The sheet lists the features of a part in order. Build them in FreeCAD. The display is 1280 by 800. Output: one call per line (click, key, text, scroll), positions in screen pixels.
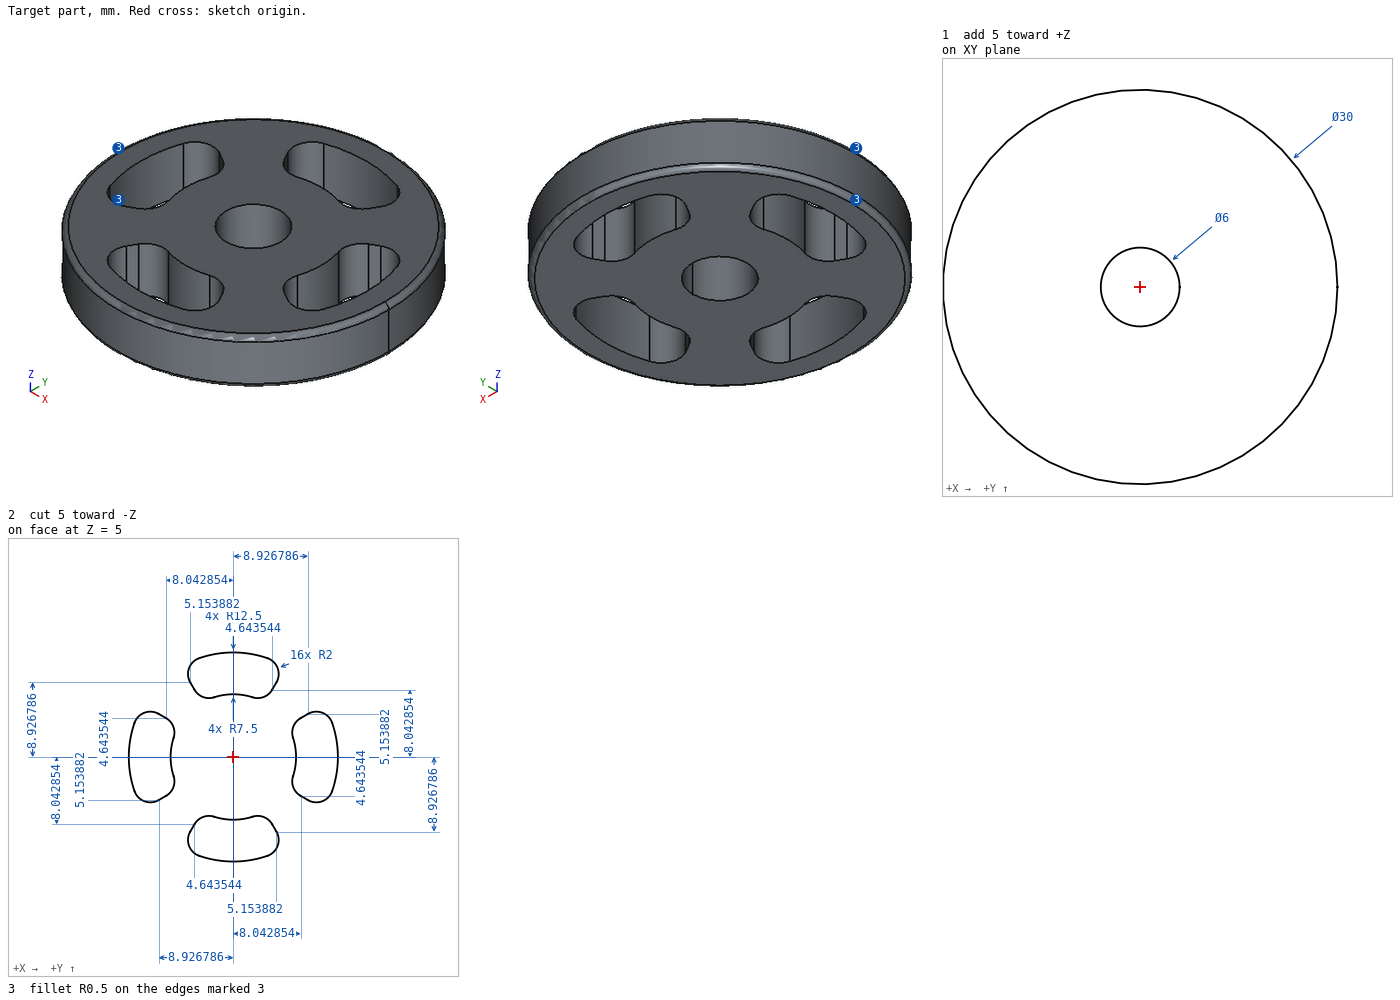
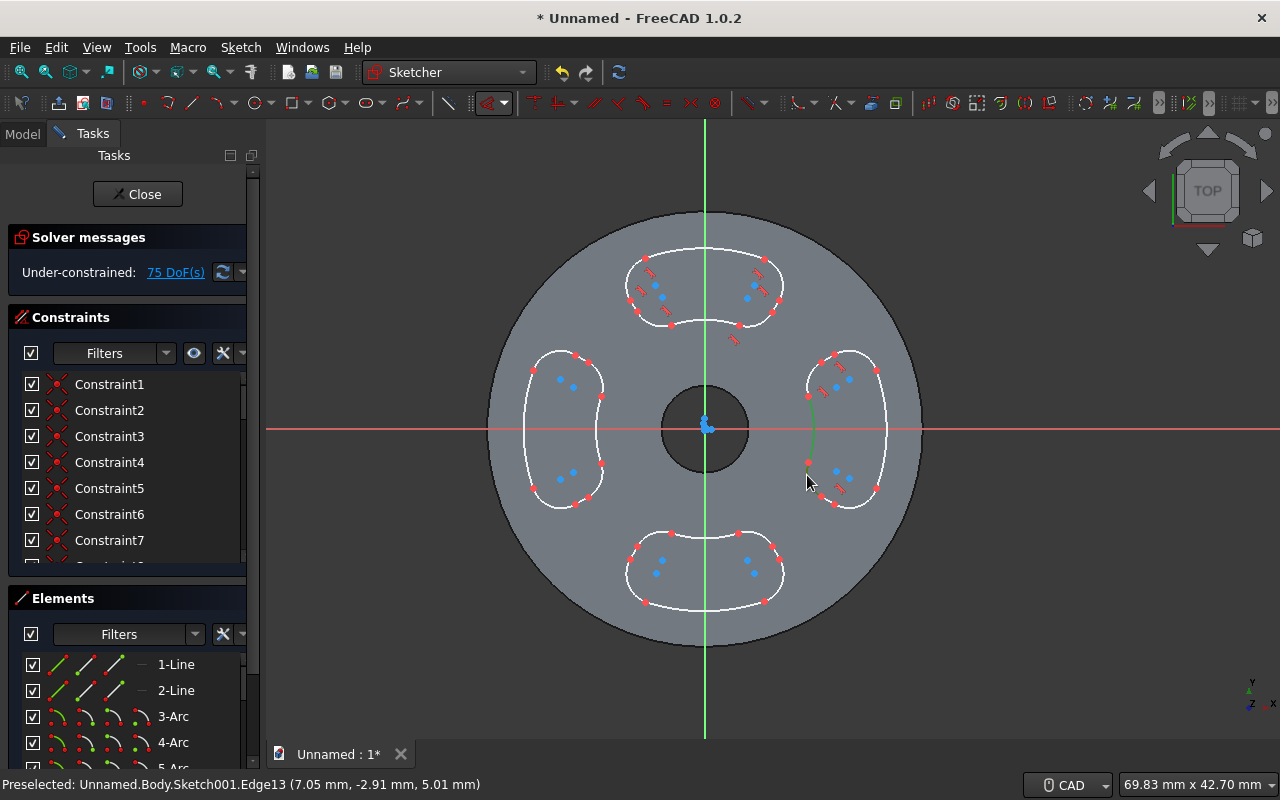
click(644, 104)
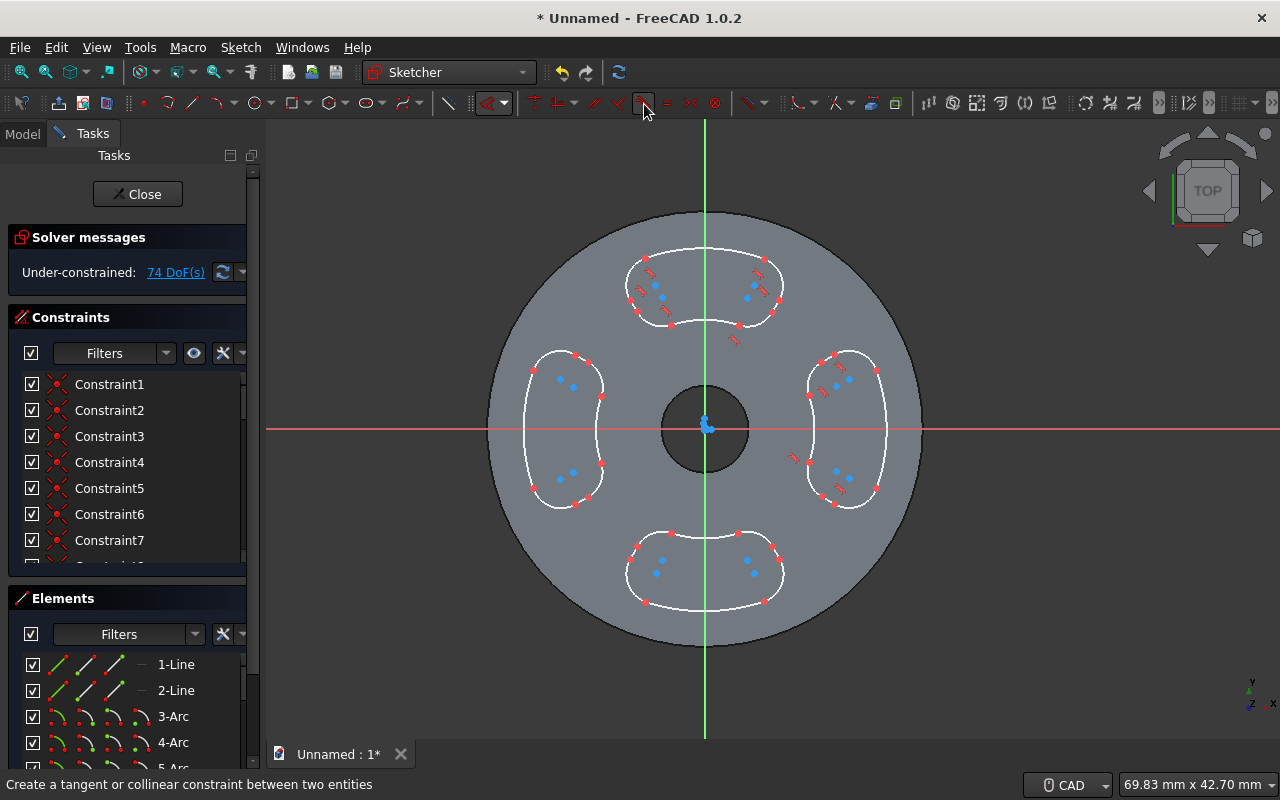
click(849, 508)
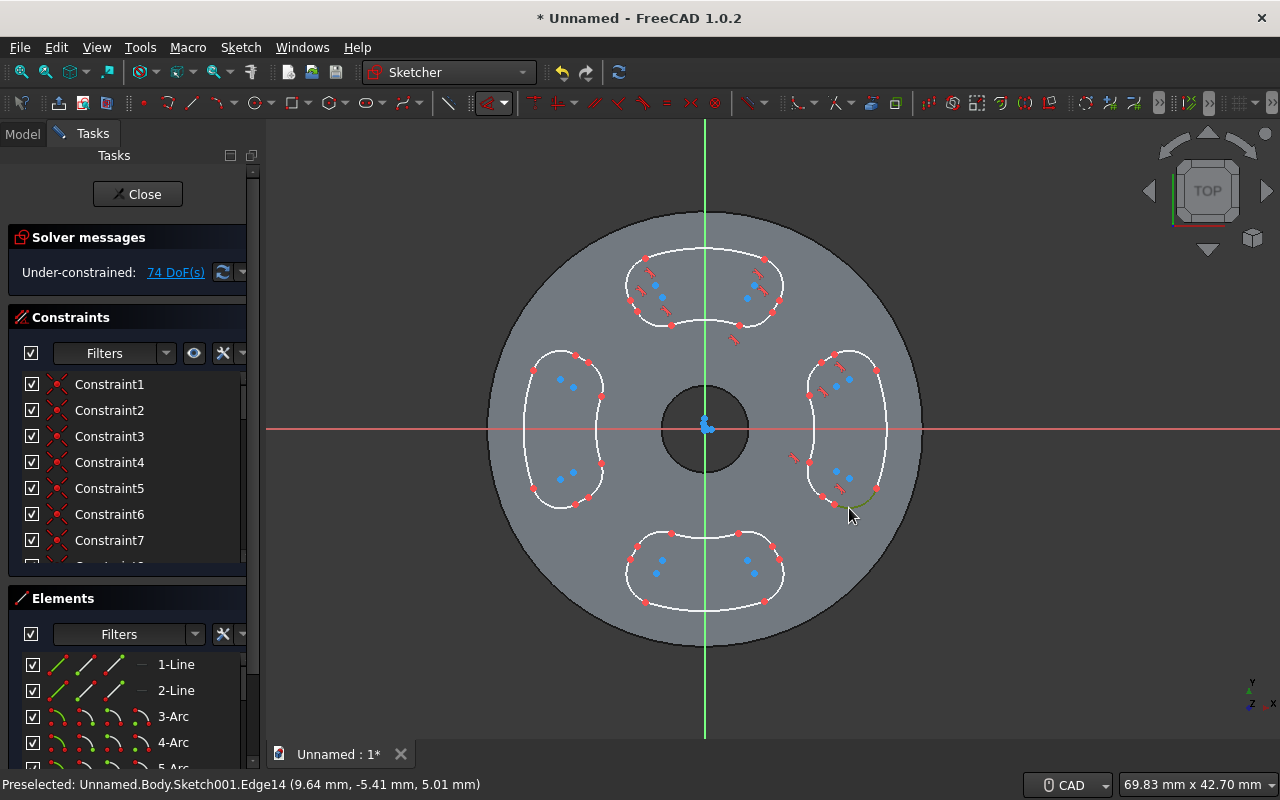
click(885, 454)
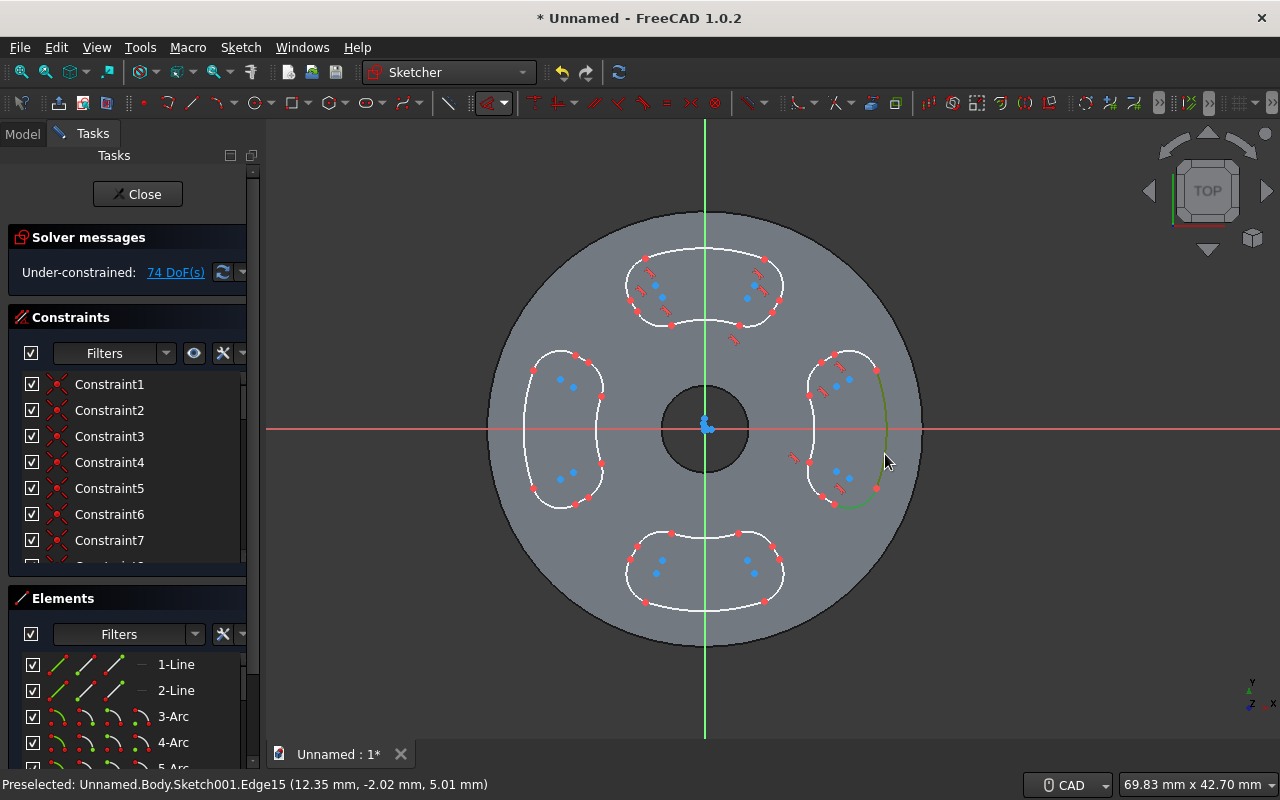
click(644, 104)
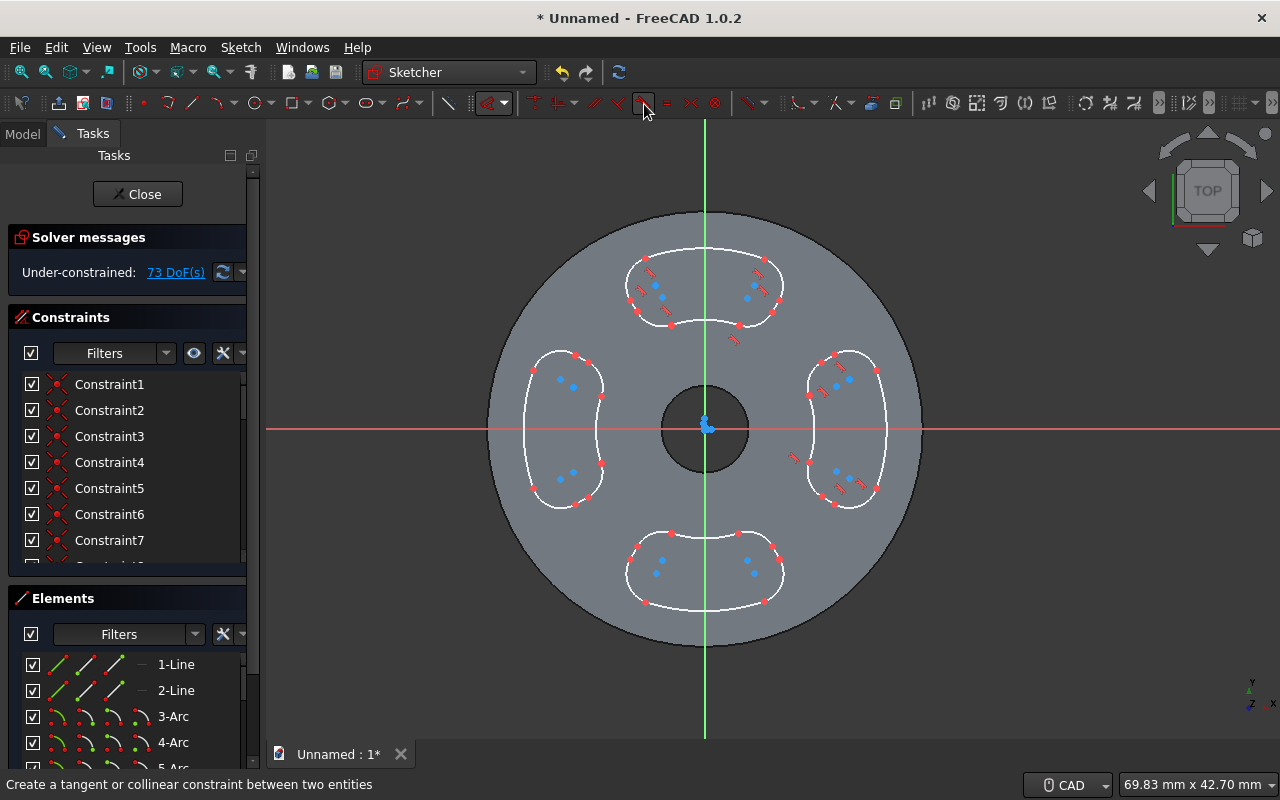
click(885, 454)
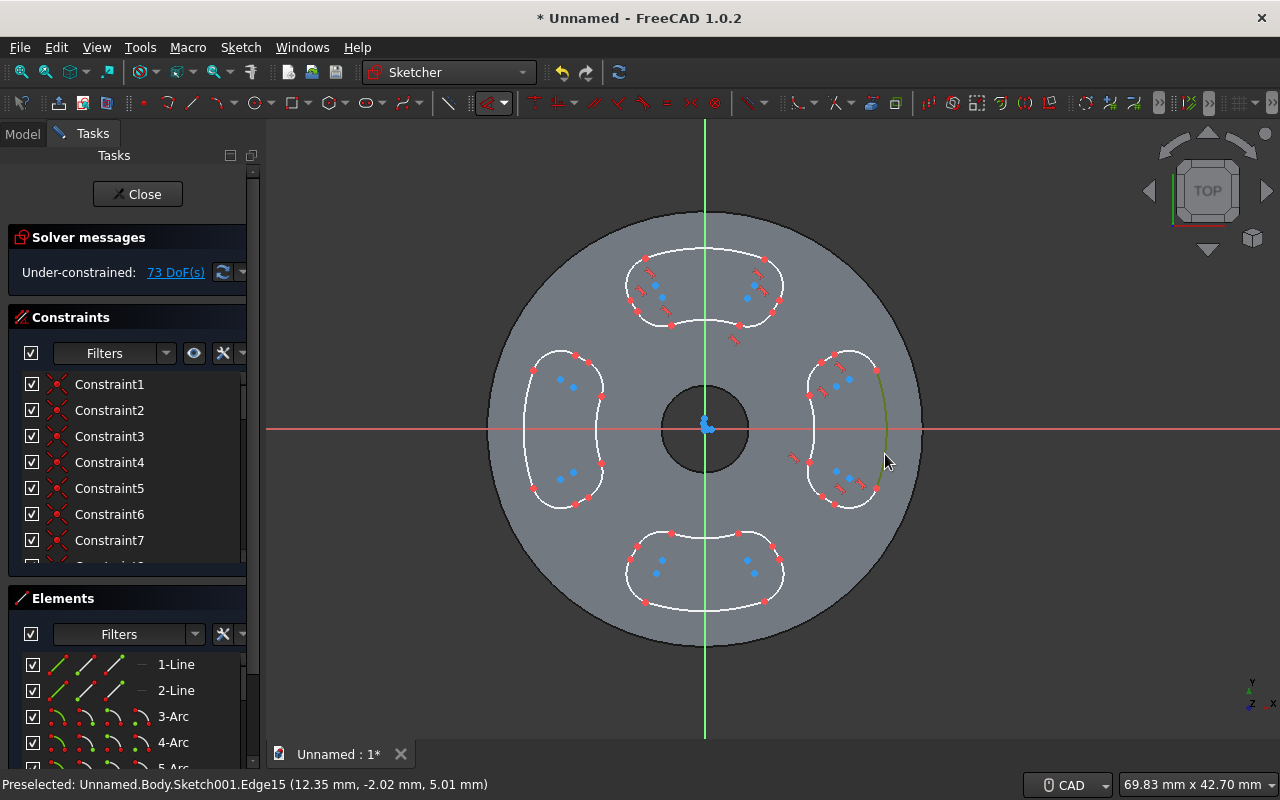
click(868, 358)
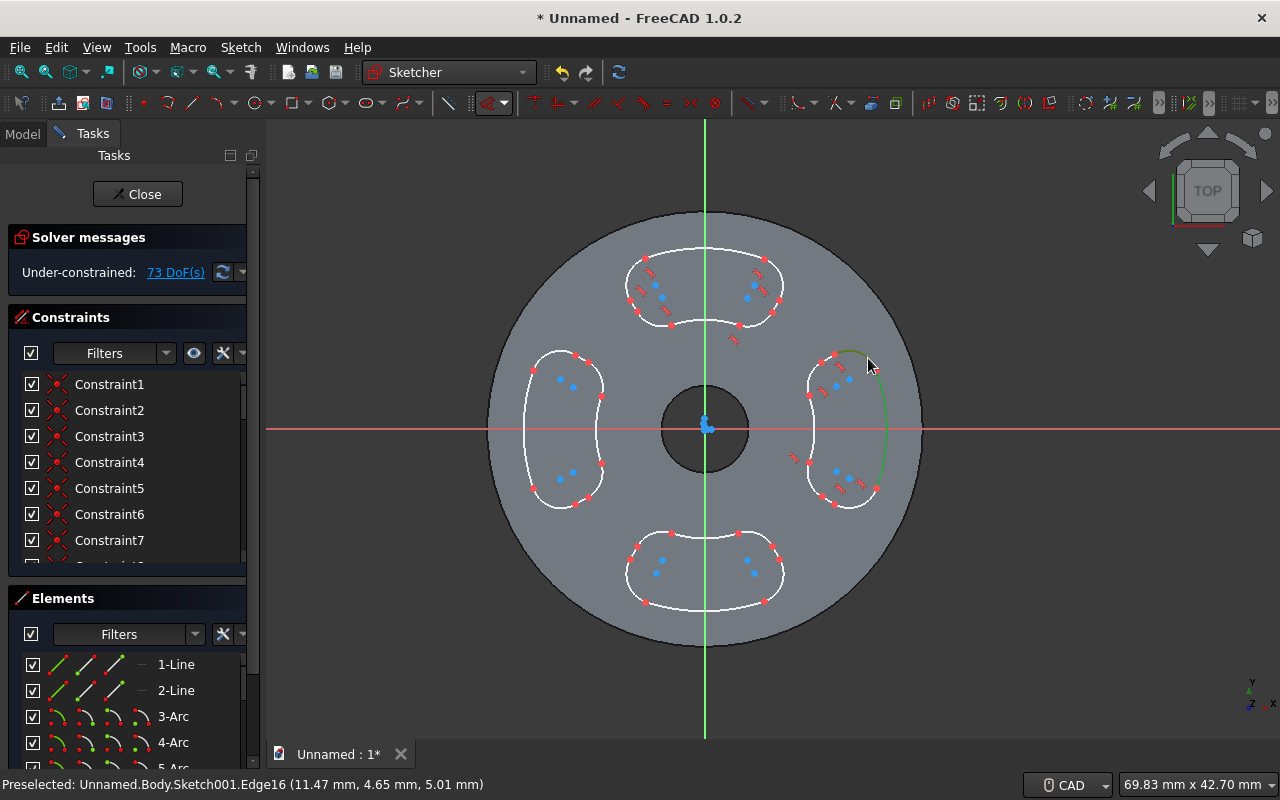
click(644, 104)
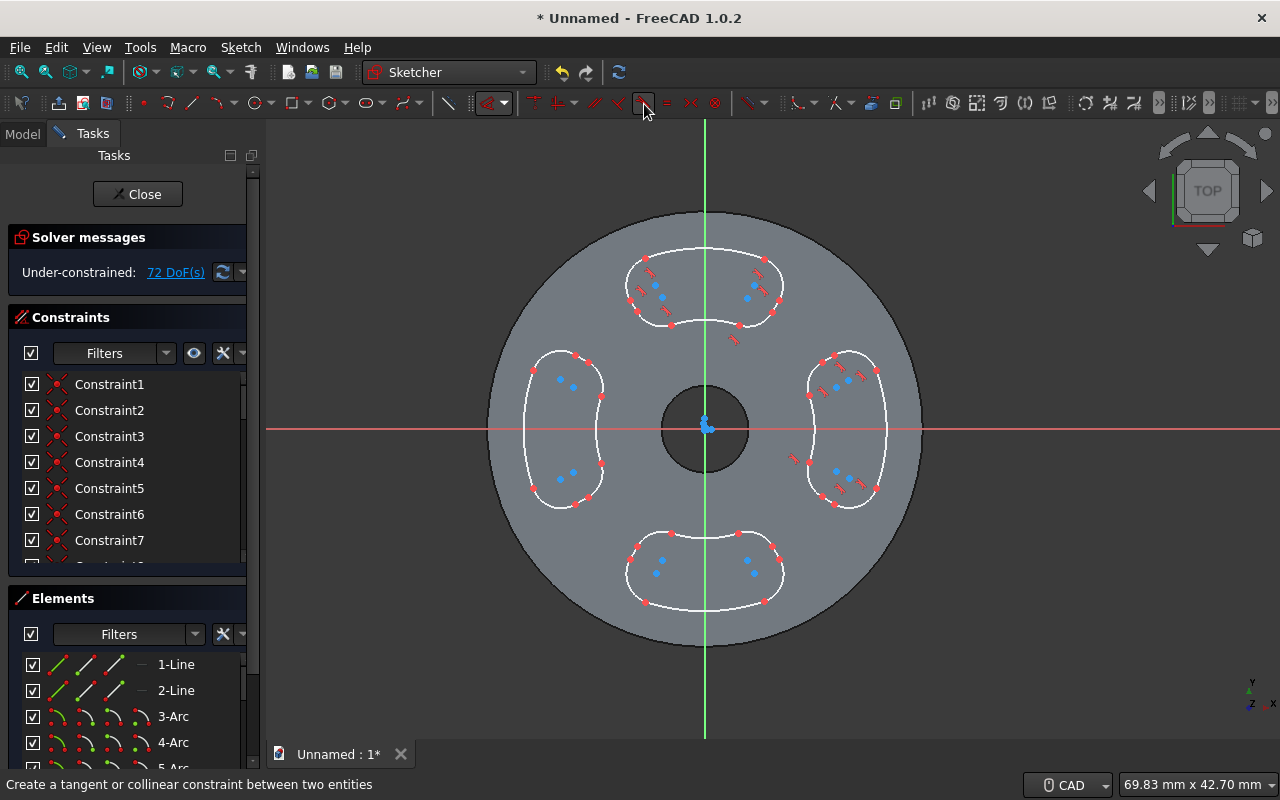
scroll(776, 553, up, 4)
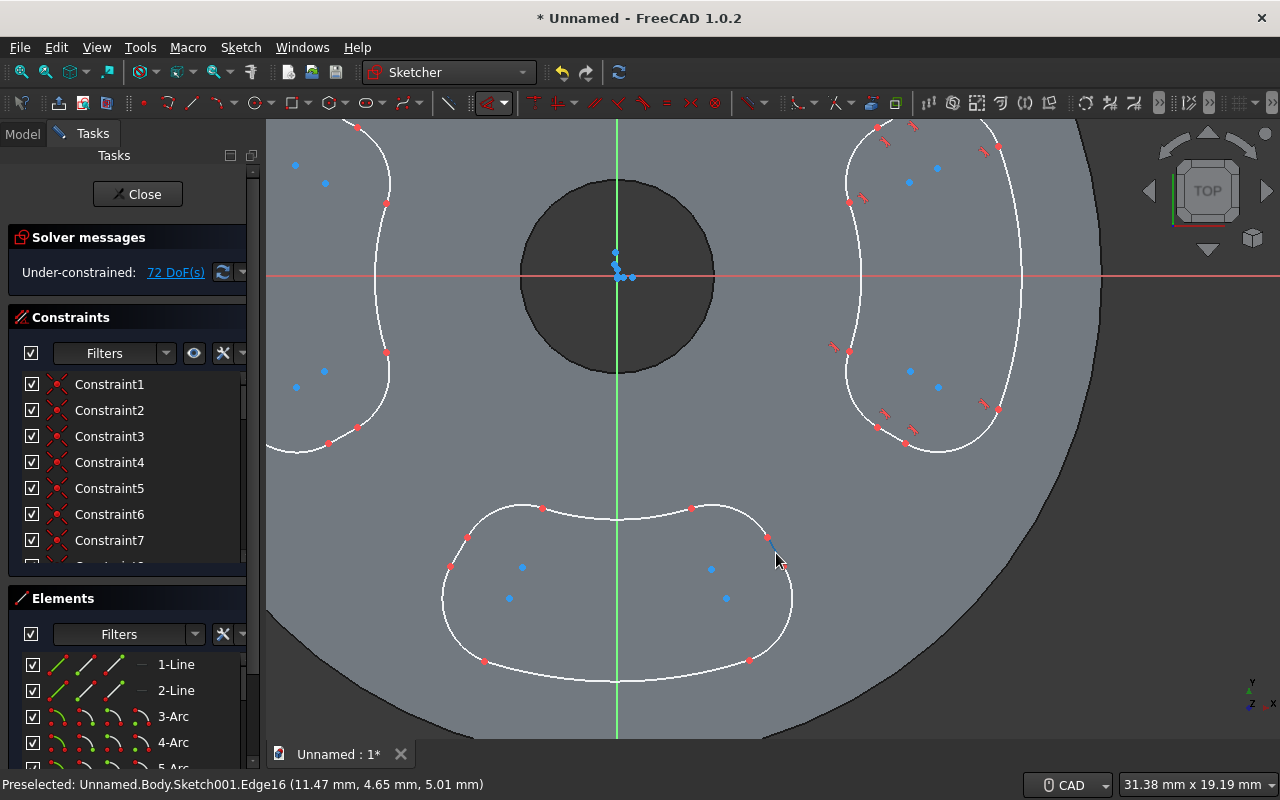
click(776, 552)